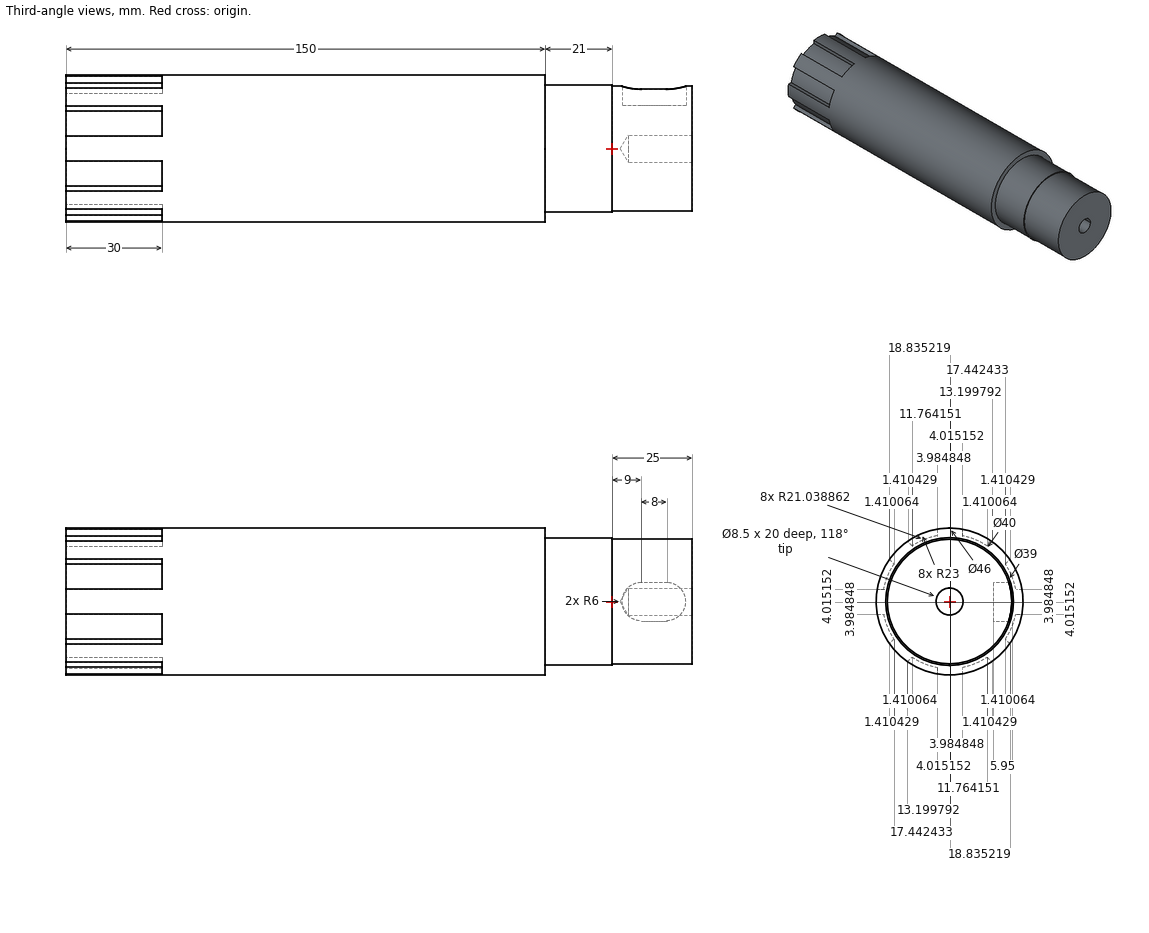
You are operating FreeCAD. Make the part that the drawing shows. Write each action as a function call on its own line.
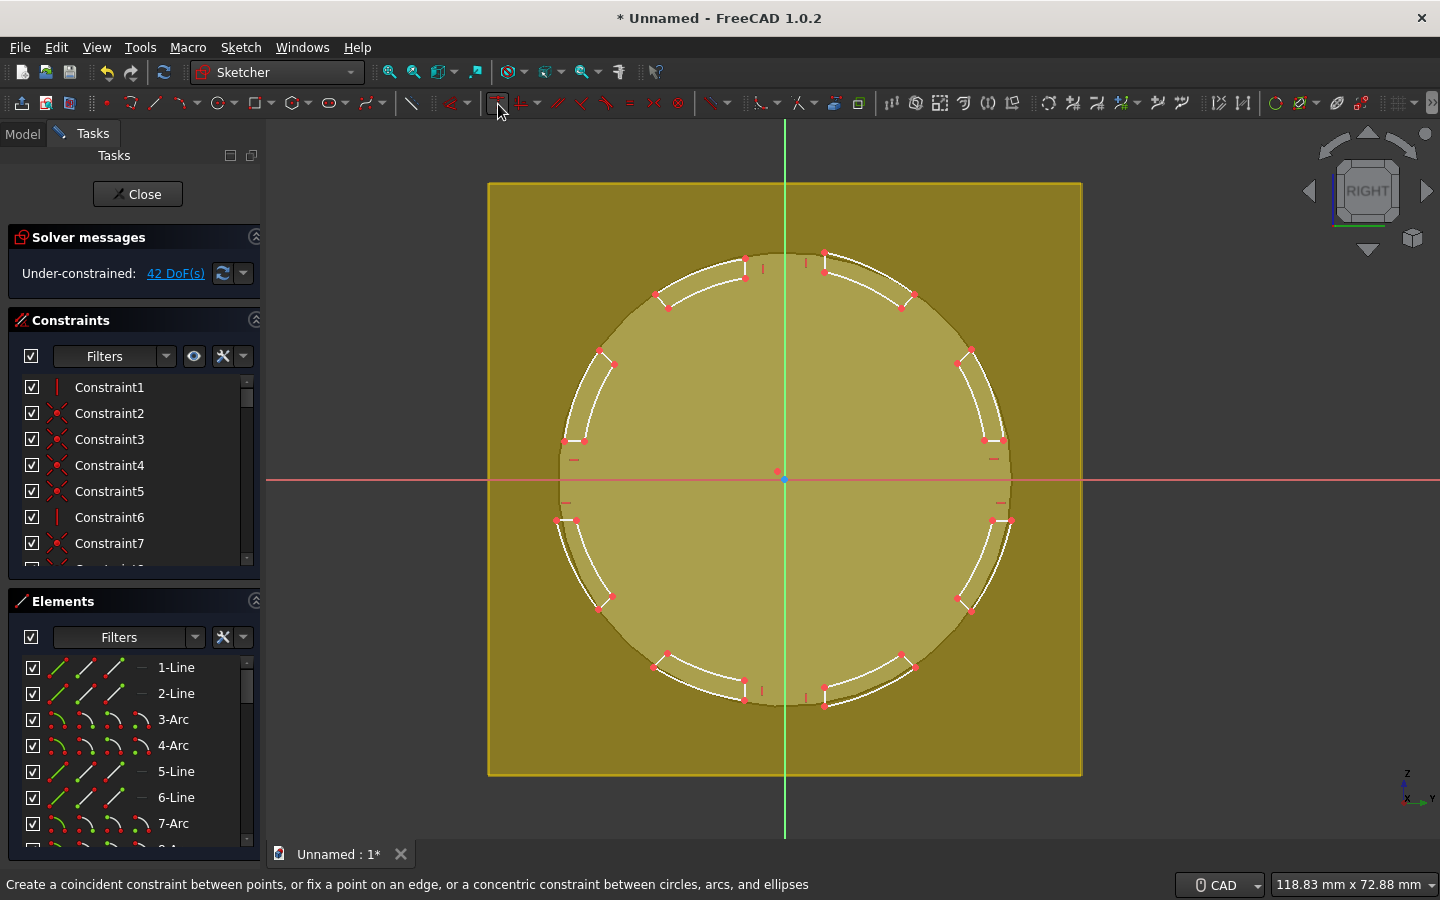
drag(767, 461, 795, 490)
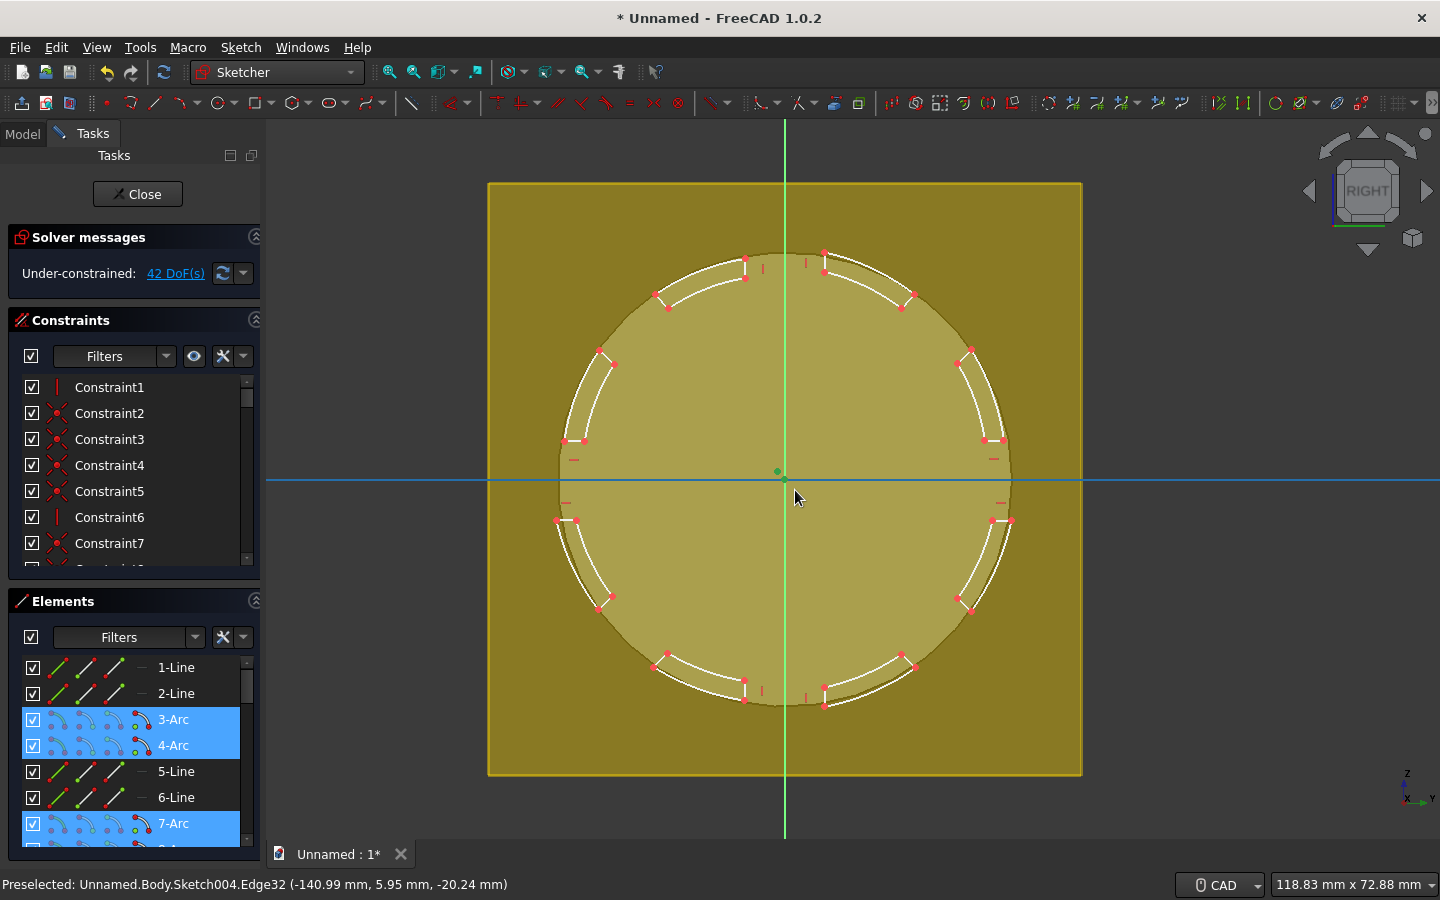
click(498, 104)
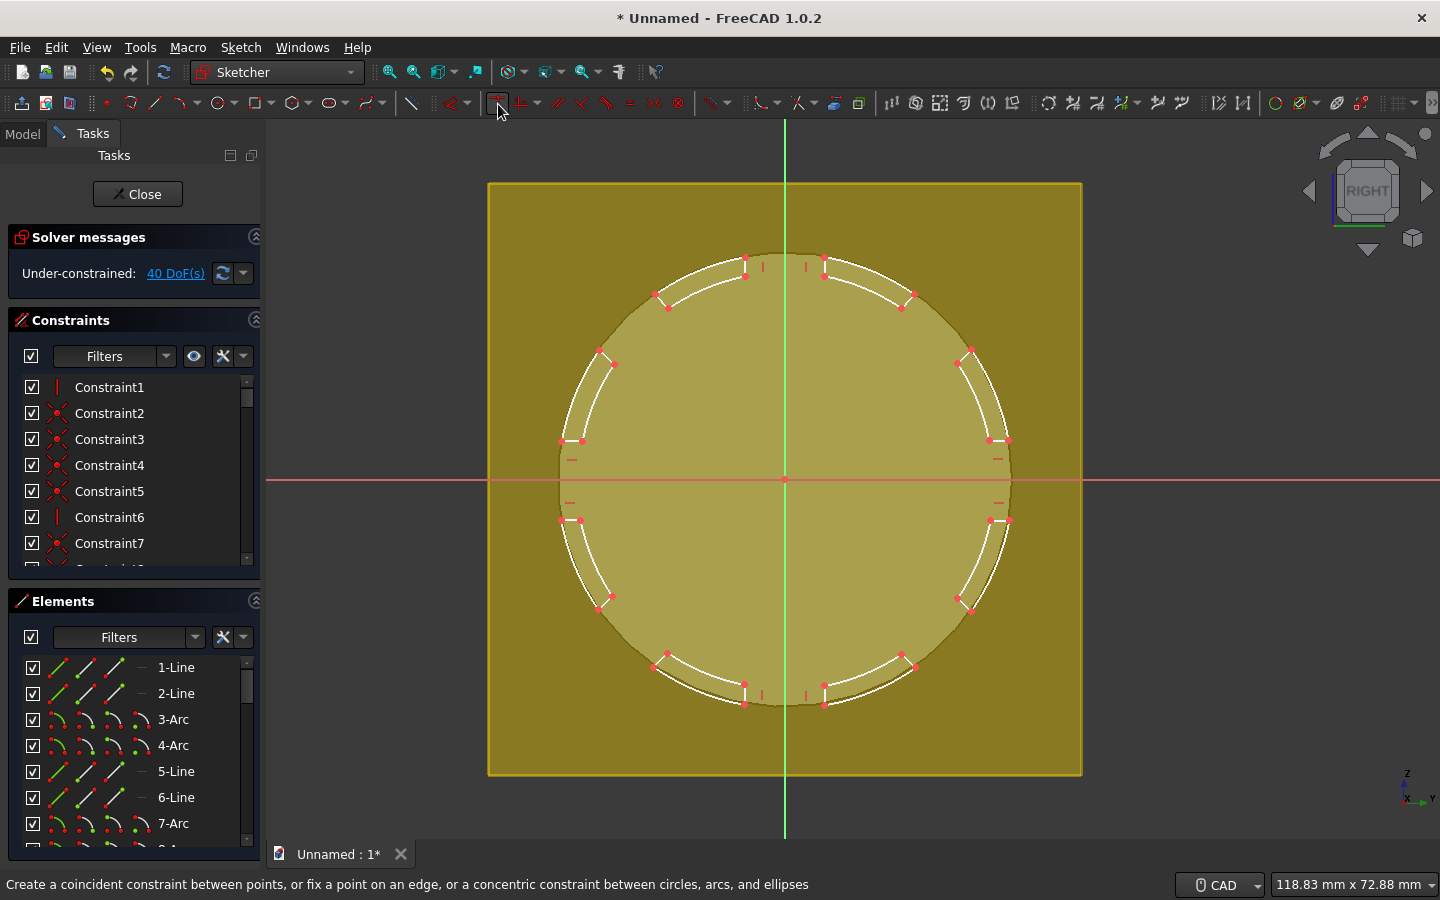
click(721, 283)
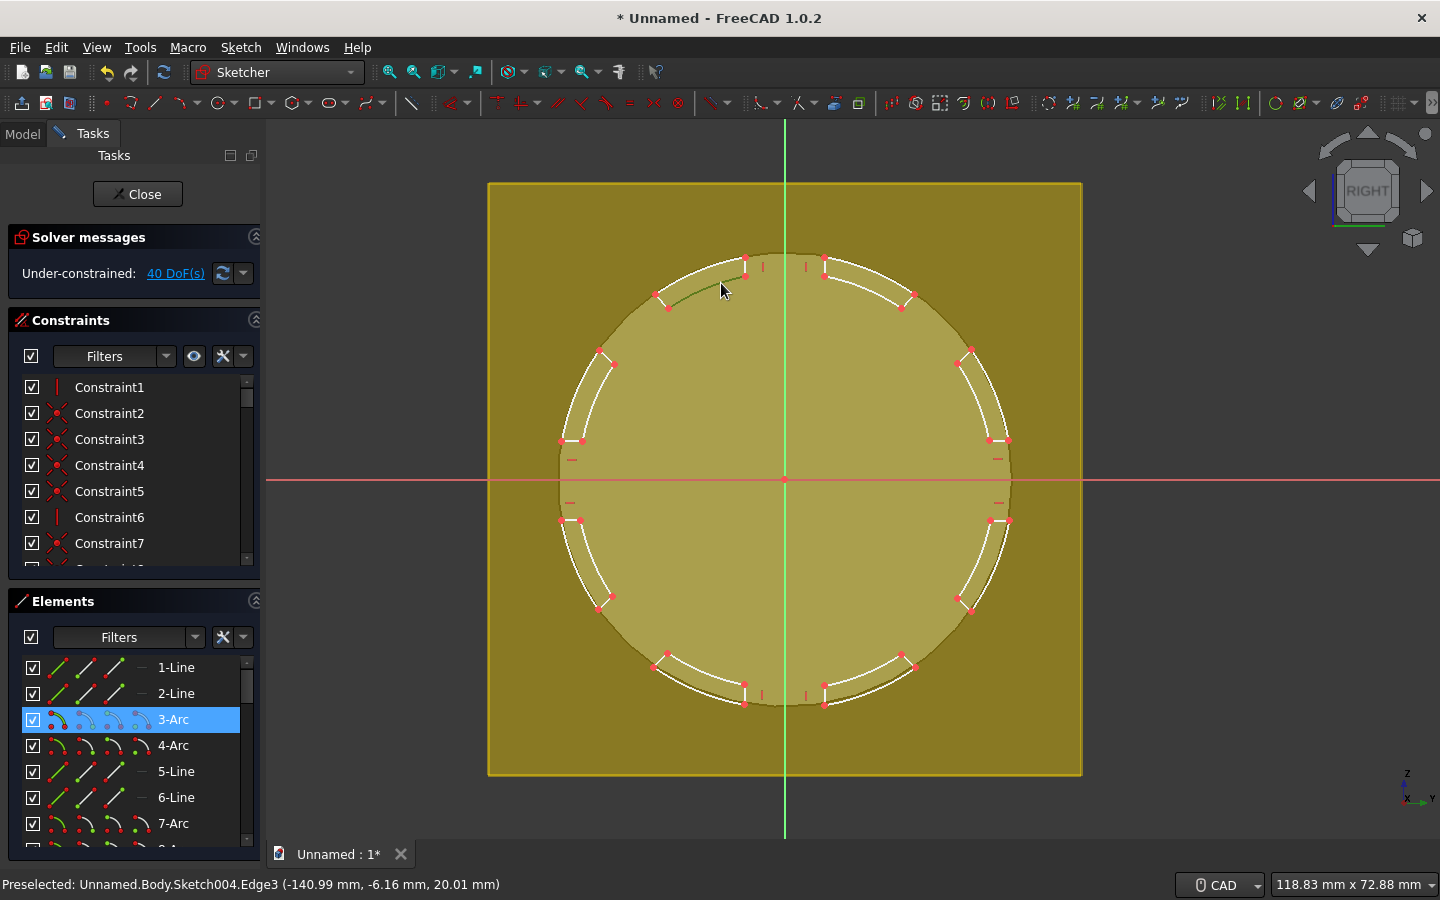
click(880, 296)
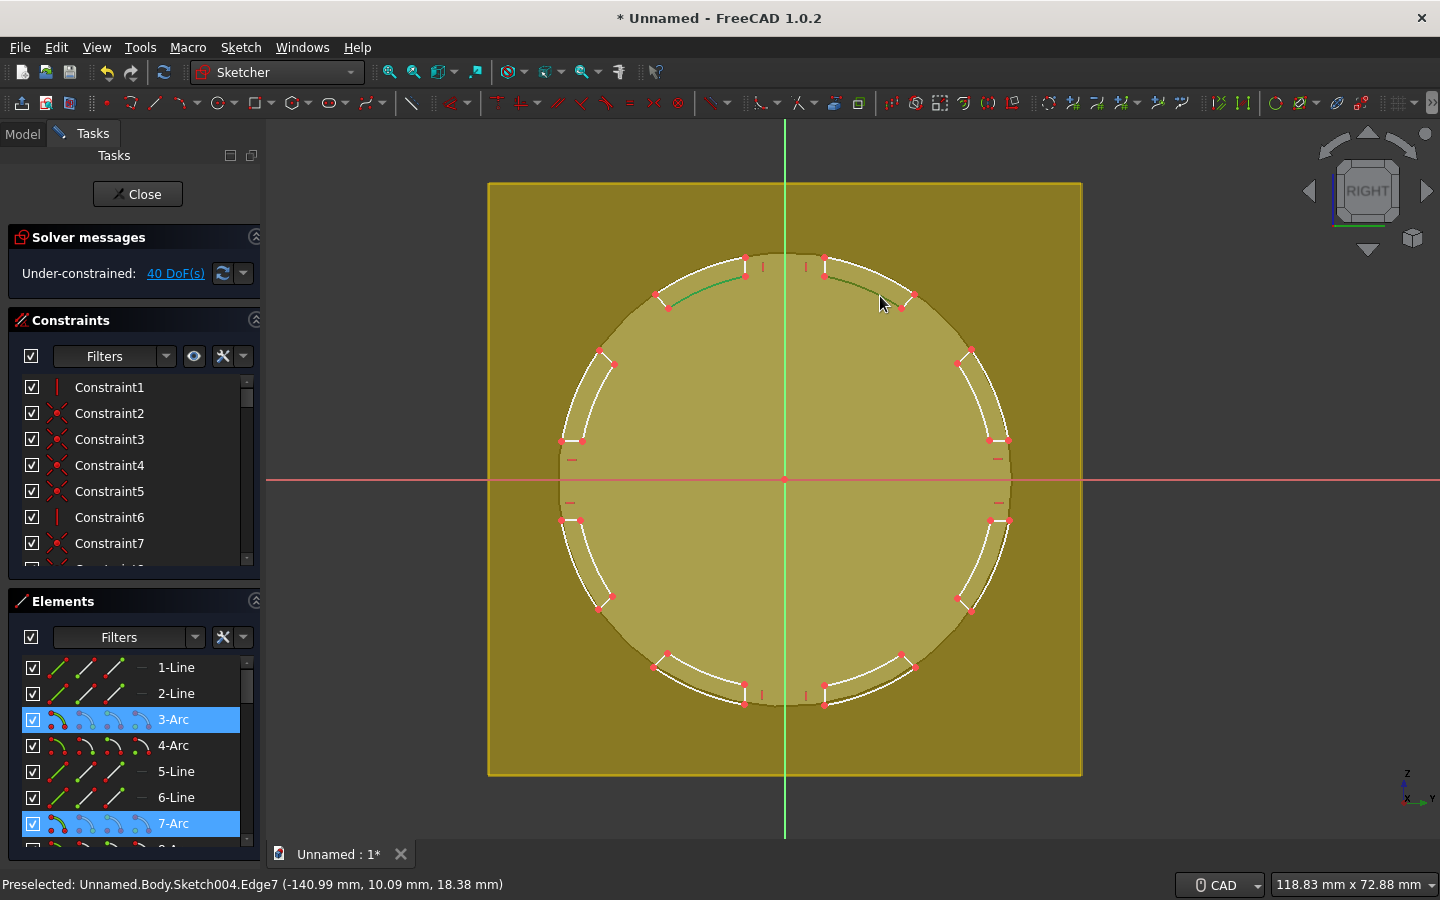
click(689, 666)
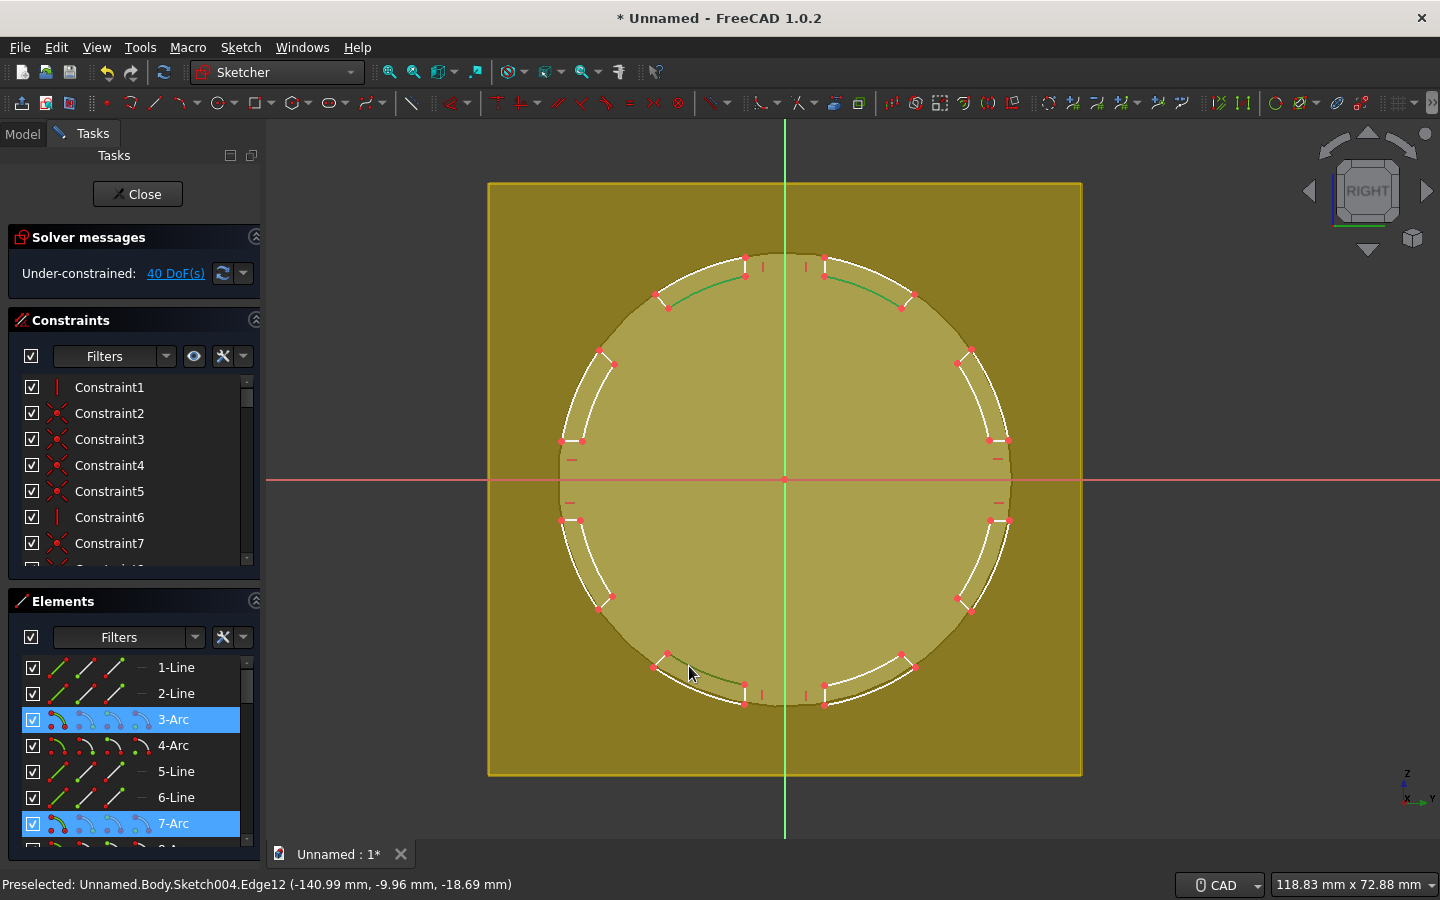
click(587, 544)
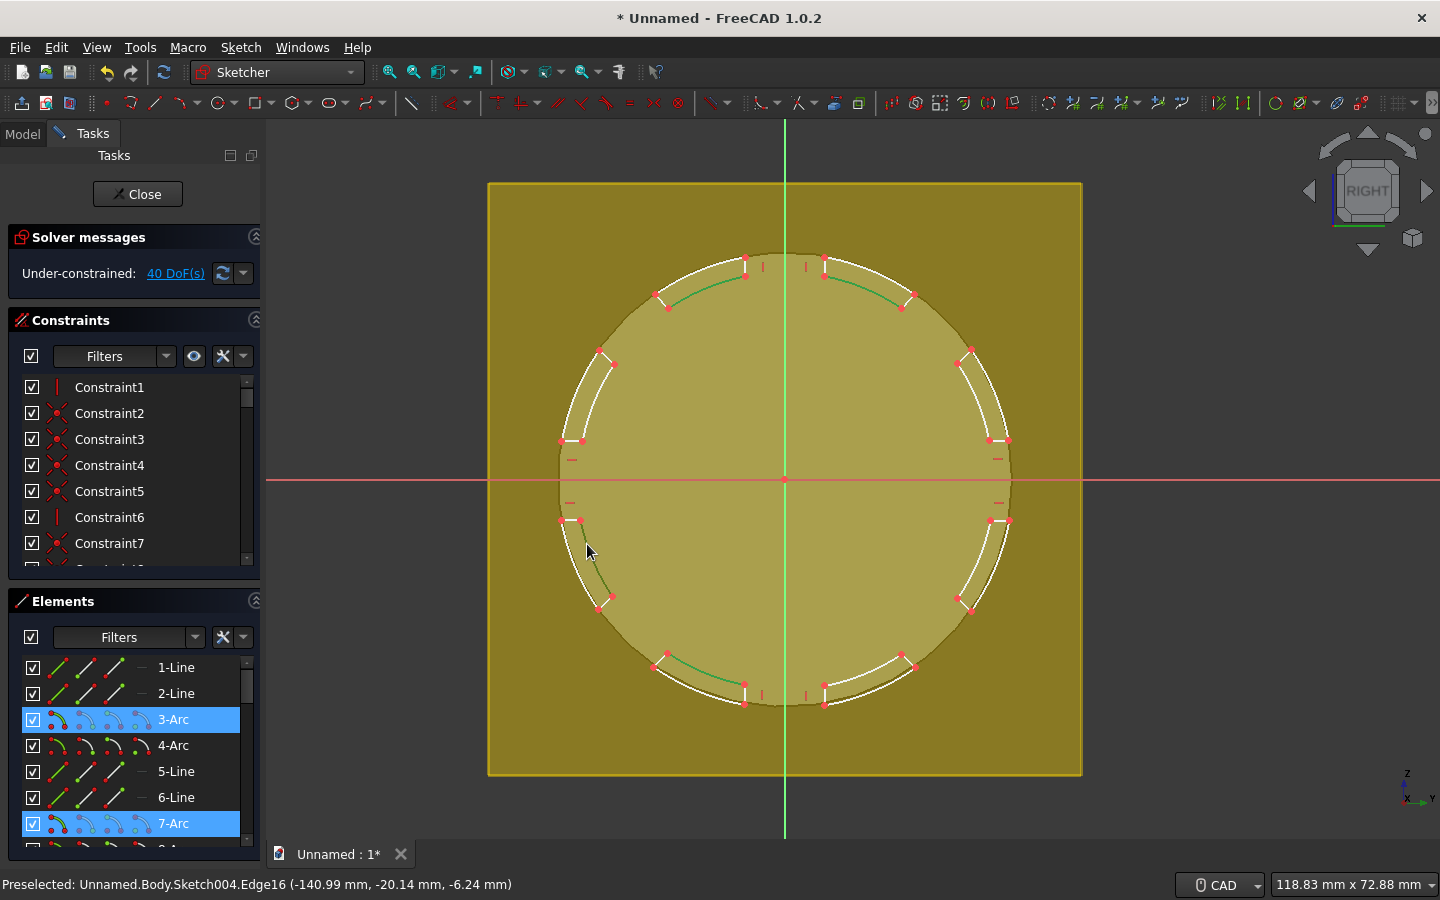
click(601, 386)